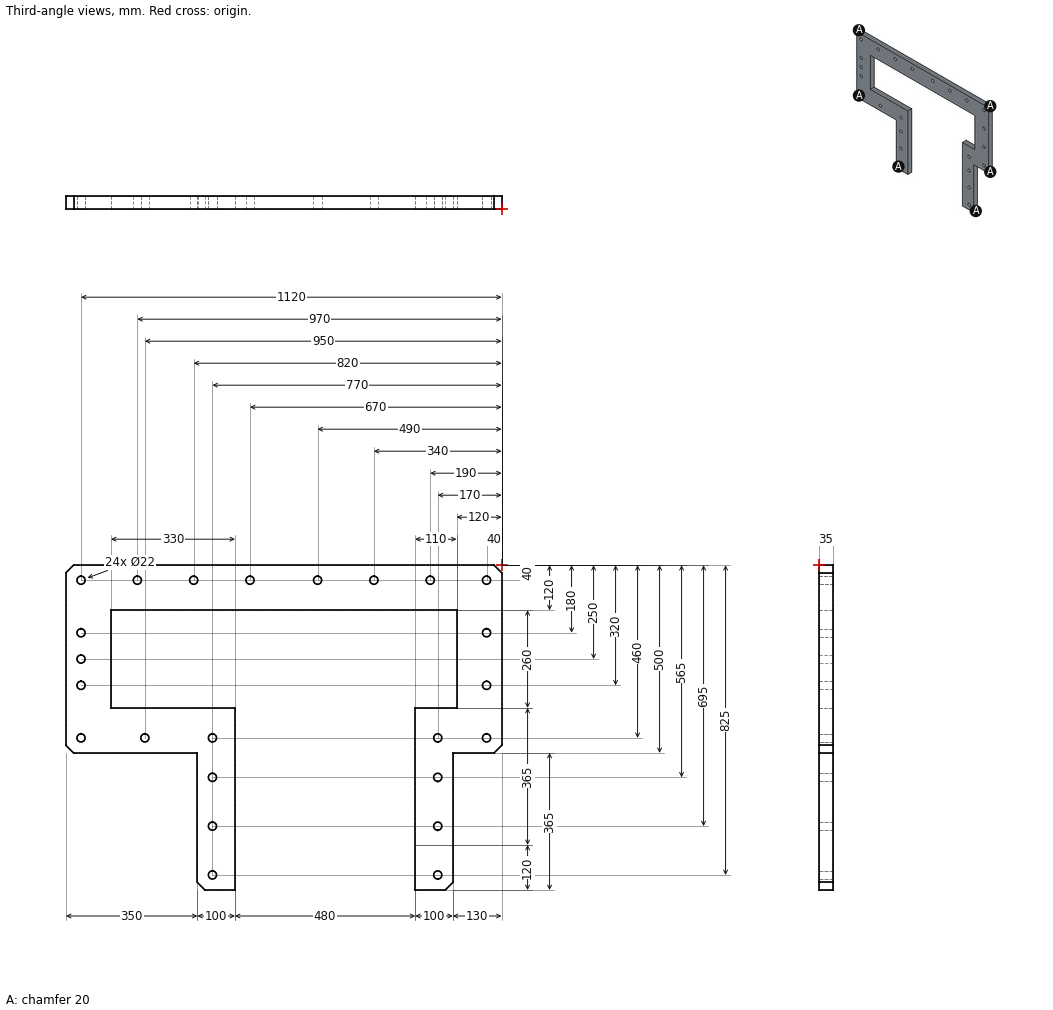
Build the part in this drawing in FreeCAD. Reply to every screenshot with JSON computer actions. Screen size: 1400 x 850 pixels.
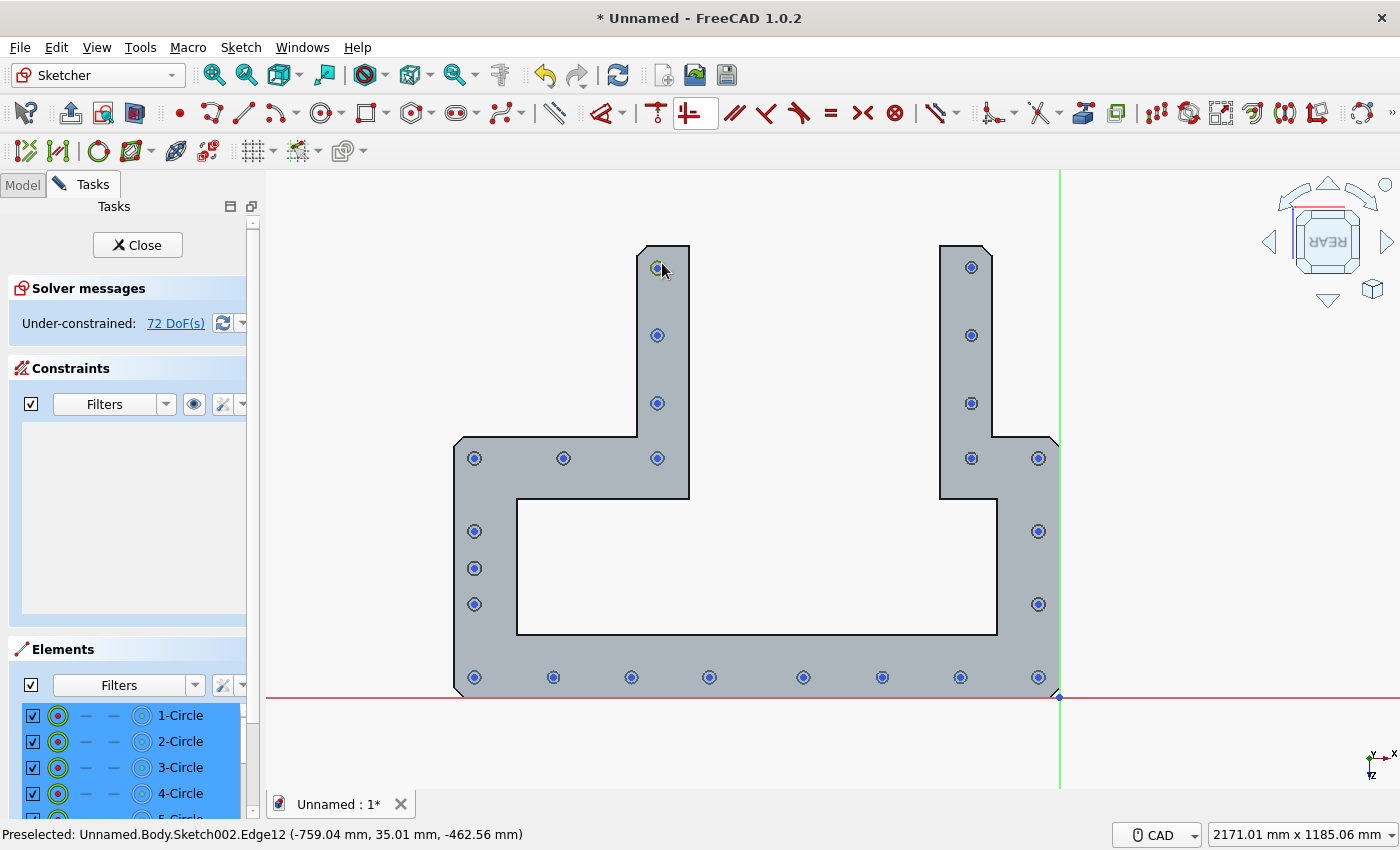
{"action": "scroll", "coordinate": [479, 600], "scroll_direction": "up", "scroll_amount": 4}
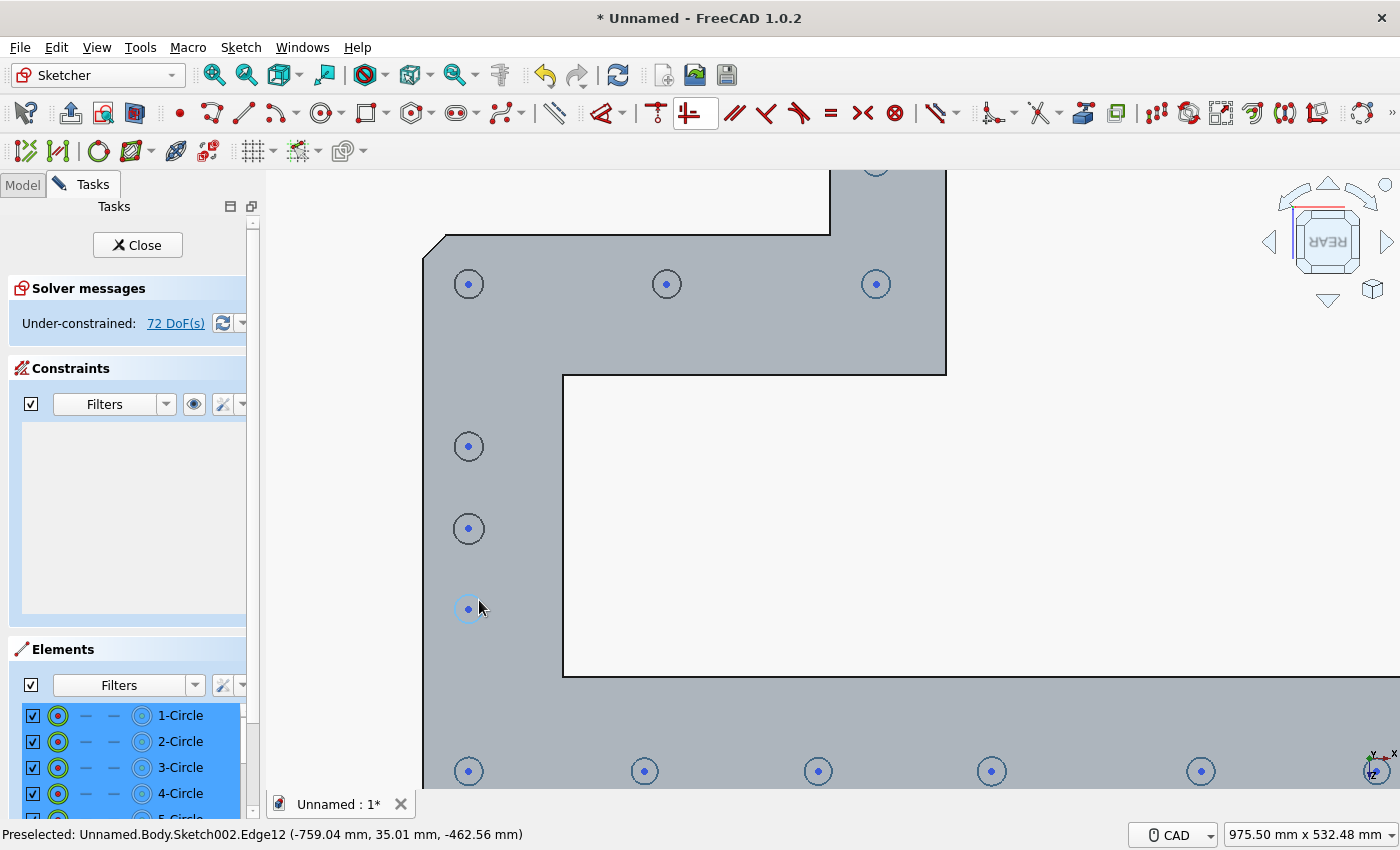
{"action": "left_click", "coordinate": [479, 599]}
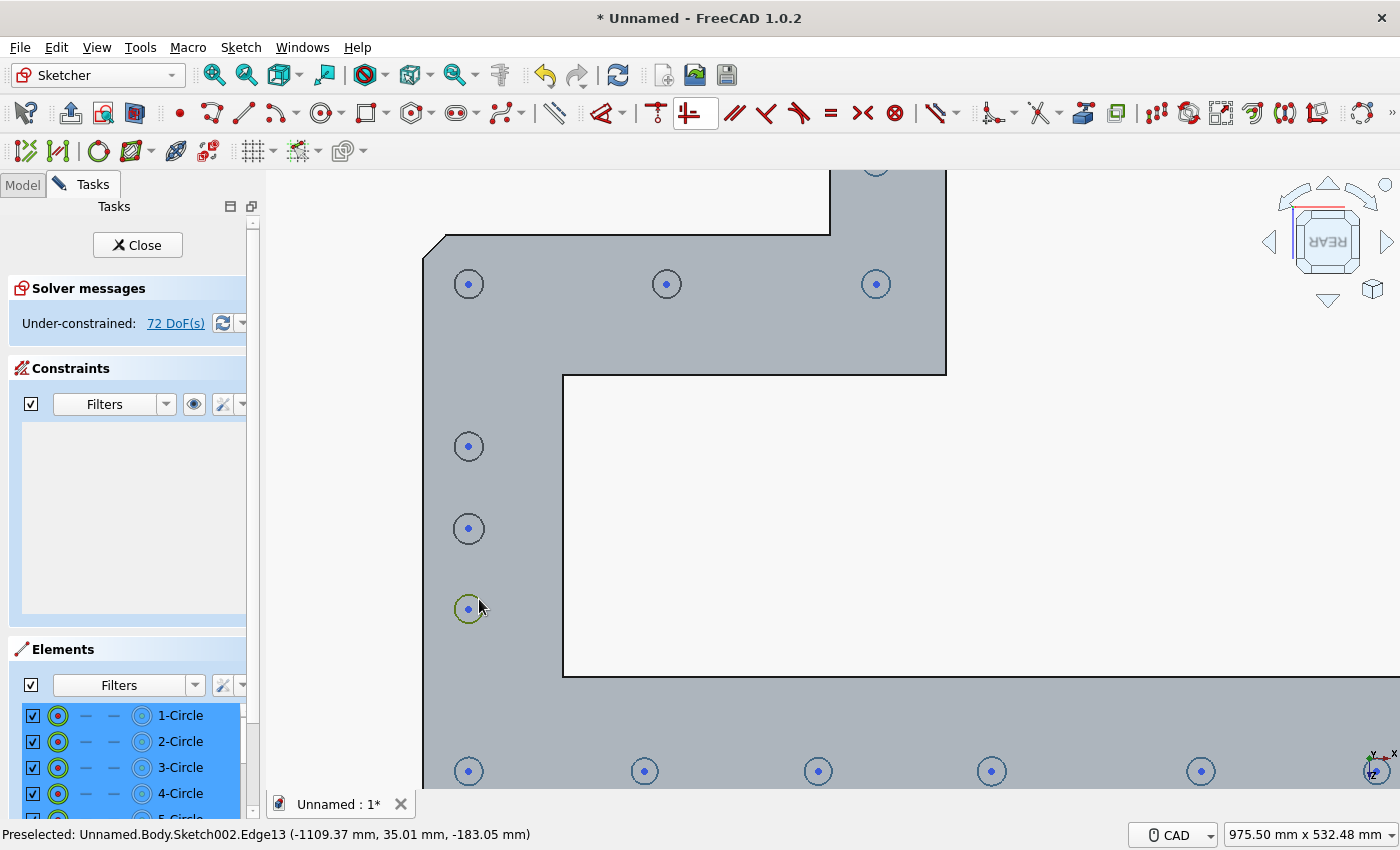
{"action": "left_click", "coordinate": [479, 518]}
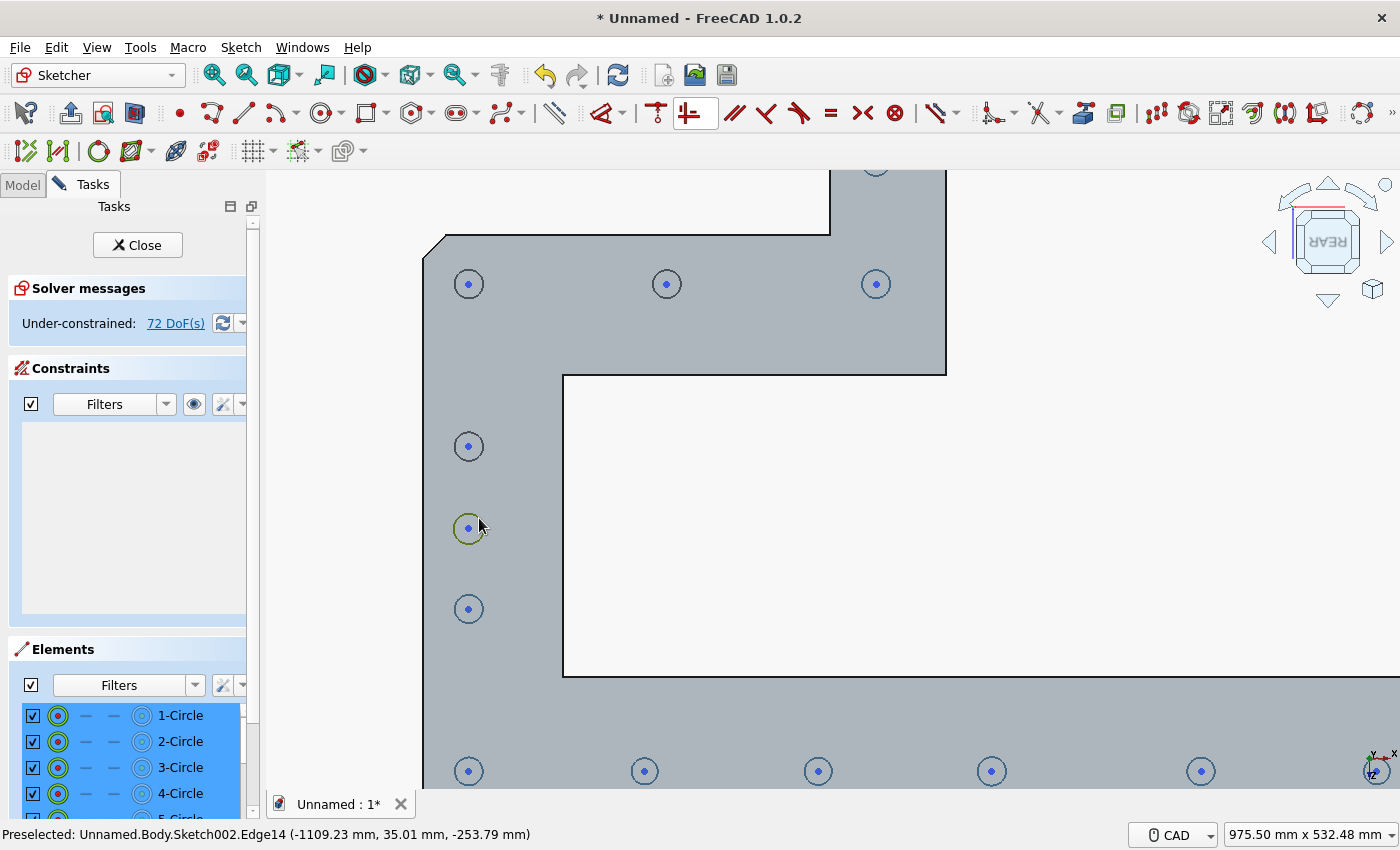
{"action": "left_click", "coordinate": [479, 437]}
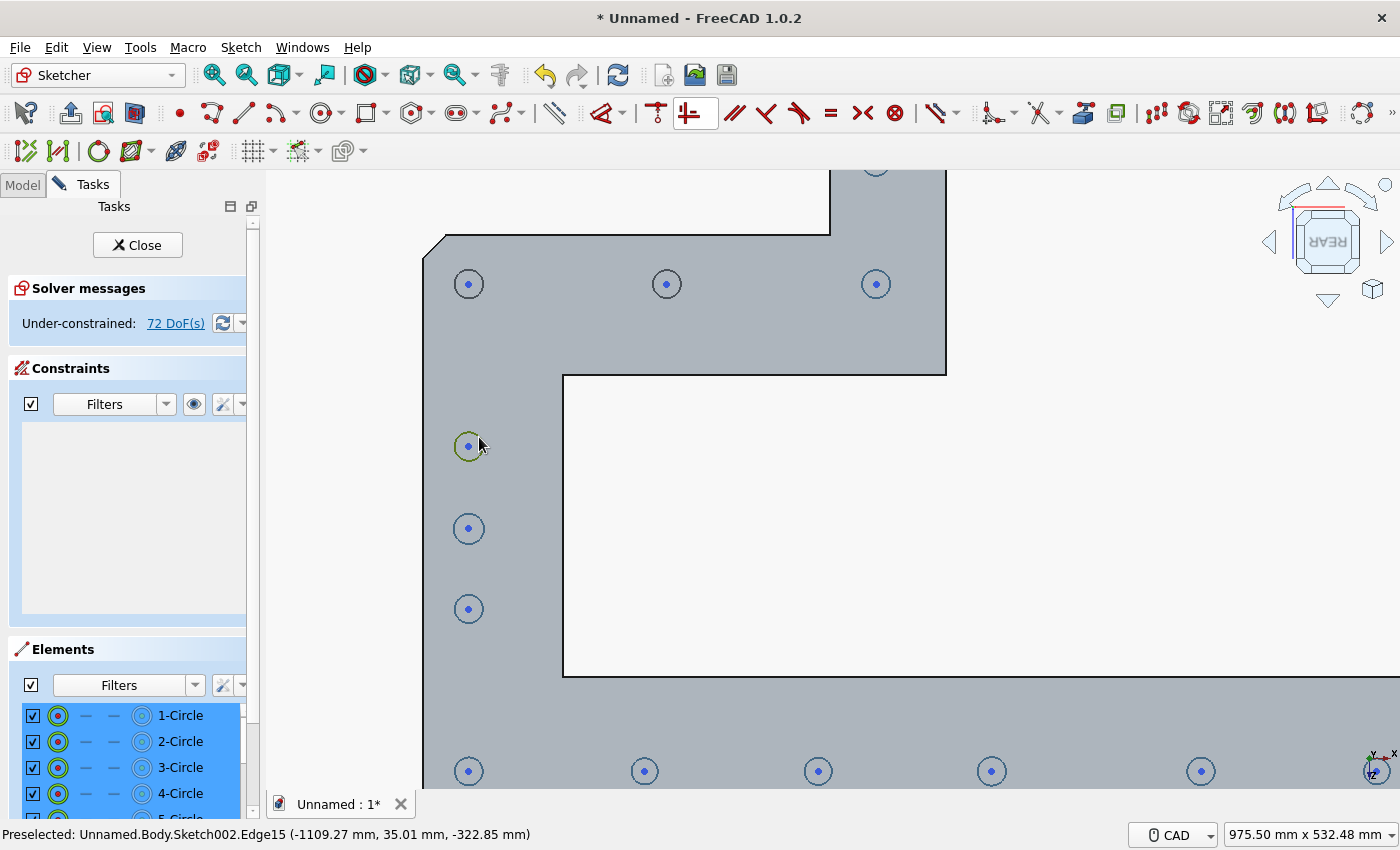
{"action": "left_click", "coordinate": [479, 274]}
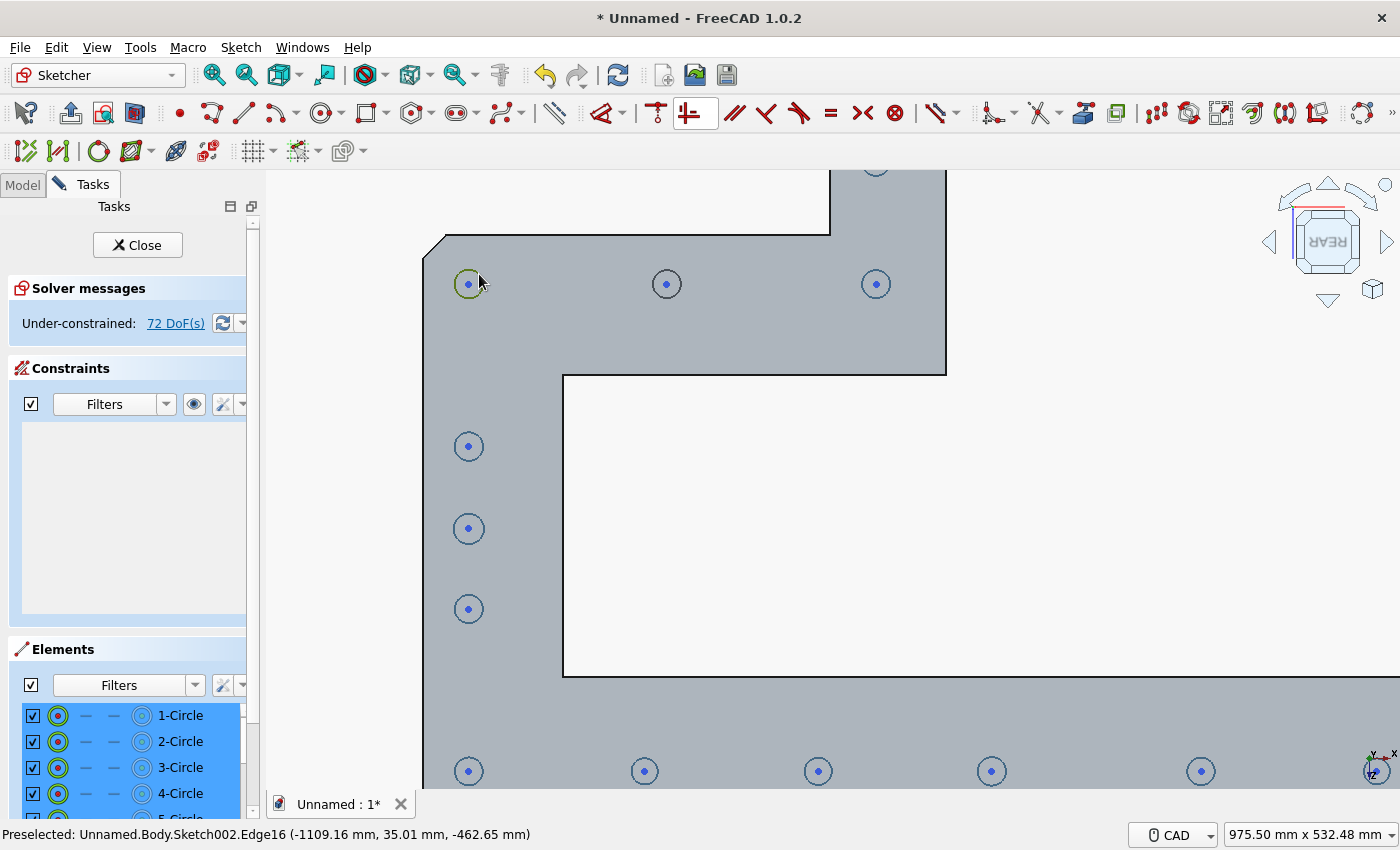
{"action": "left_click", "coordinate": [677, 274]}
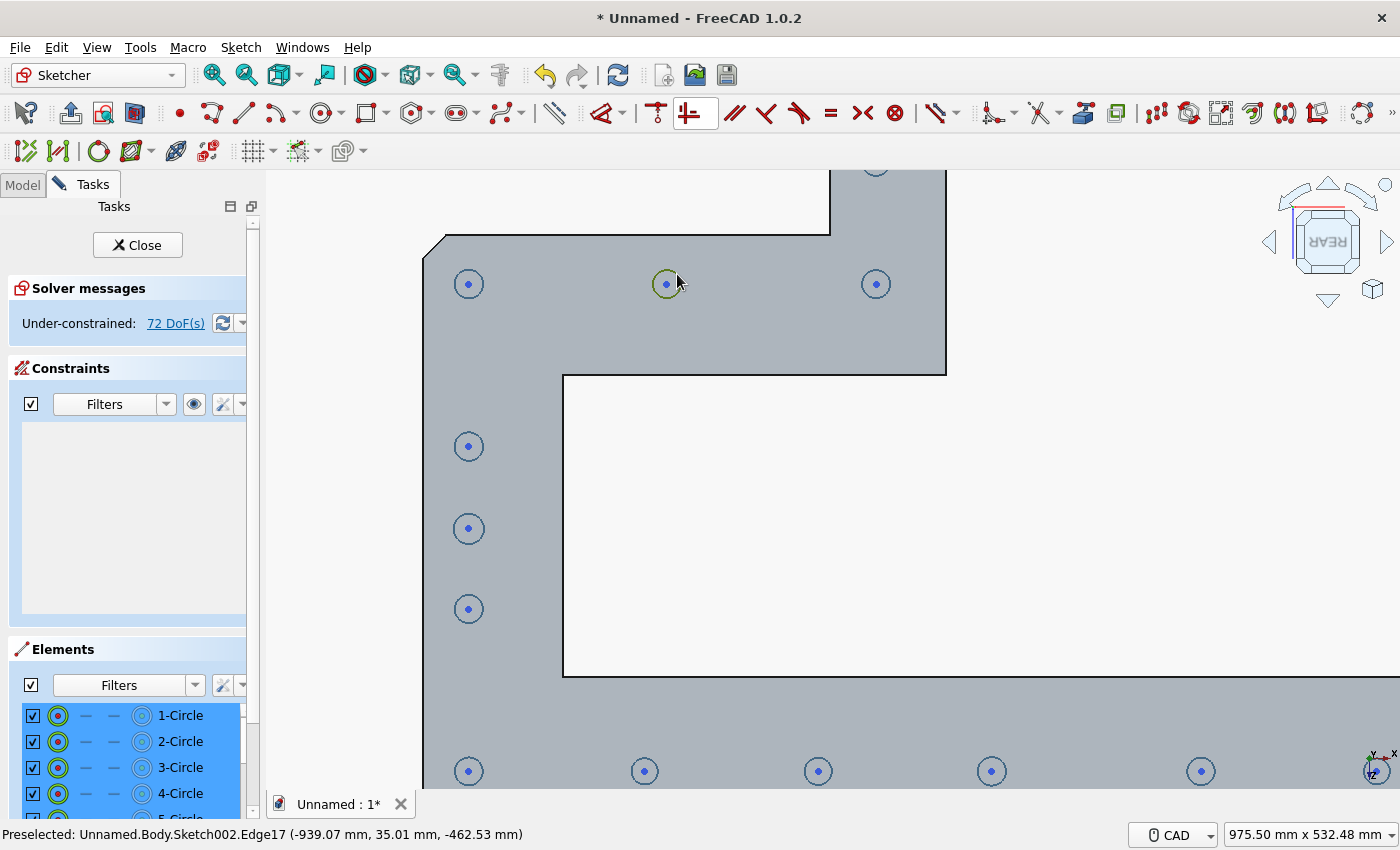
{"action": "scroll", "coordinate": [479, 601], "scroll_direction": "down", "scroll_amount": 4}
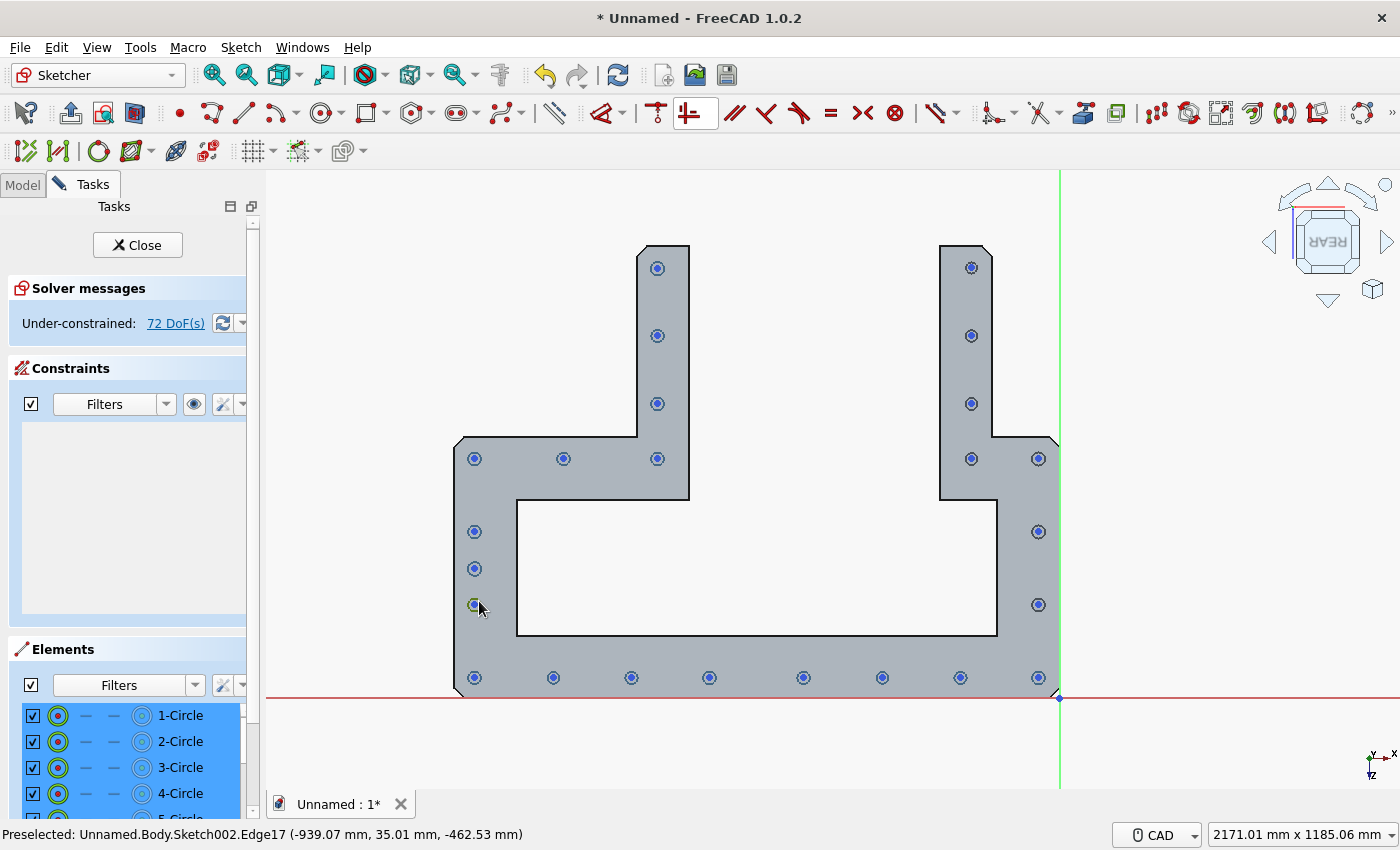
{"action": "scroll", "coordinate": [976, 455], "scroll_direction": "up", "scroll_amount": 5}